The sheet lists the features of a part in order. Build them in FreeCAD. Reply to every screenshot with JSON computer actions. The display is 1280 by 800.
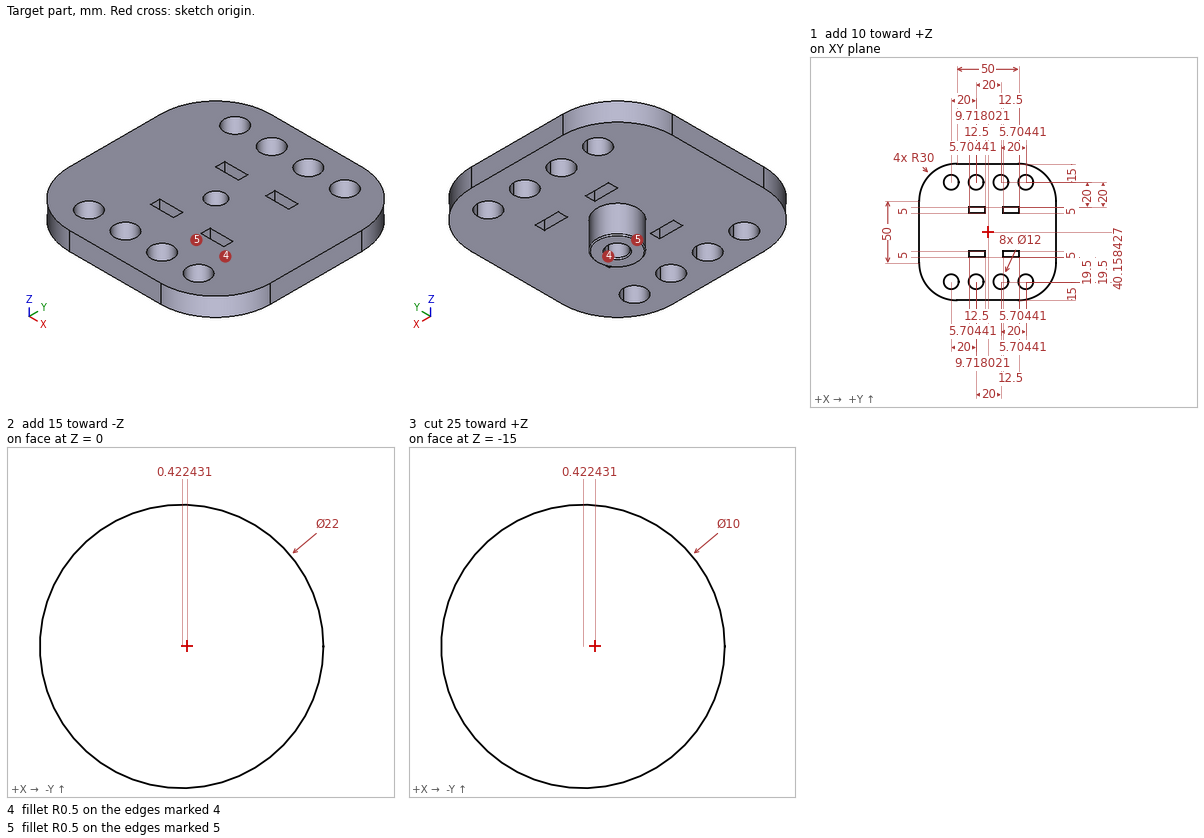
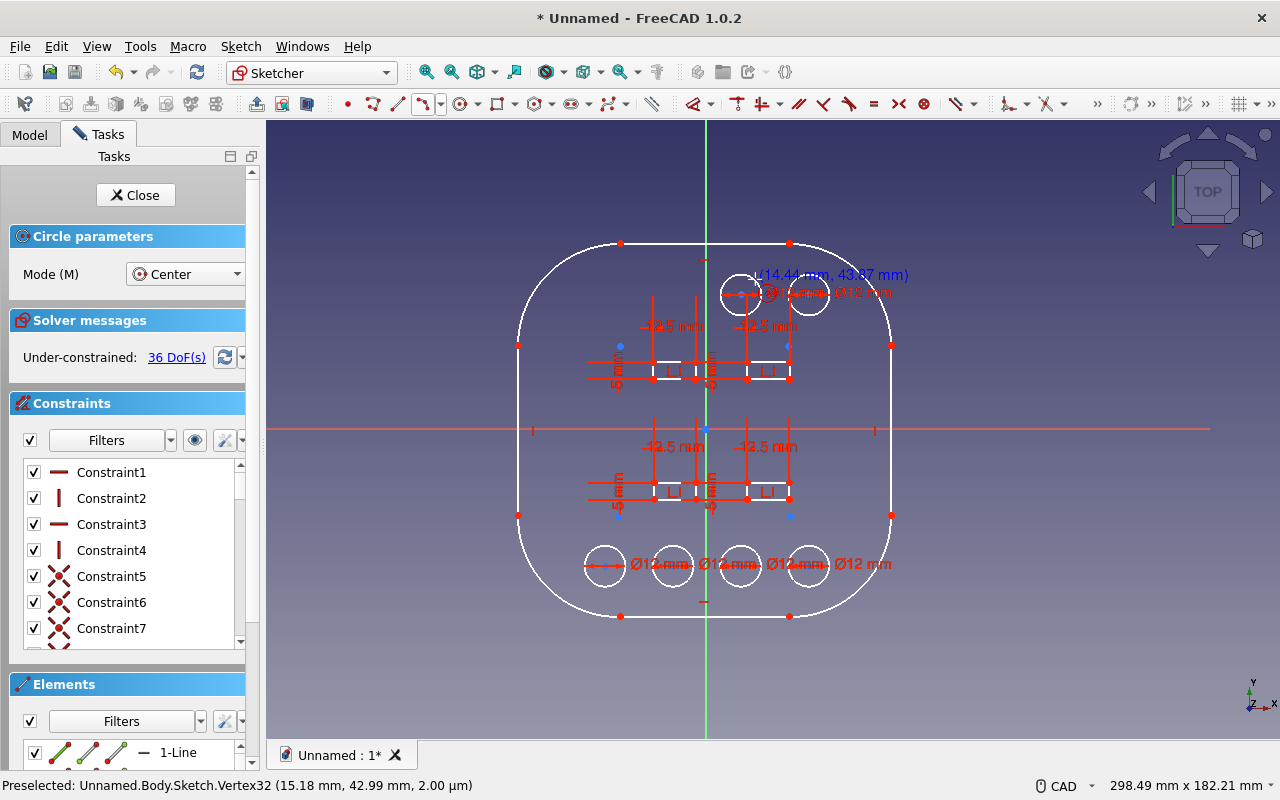
{"action": "left_click", "coordinate": [673, 294]}
{"action": "mouse_move", "coordinate": [687, 279]}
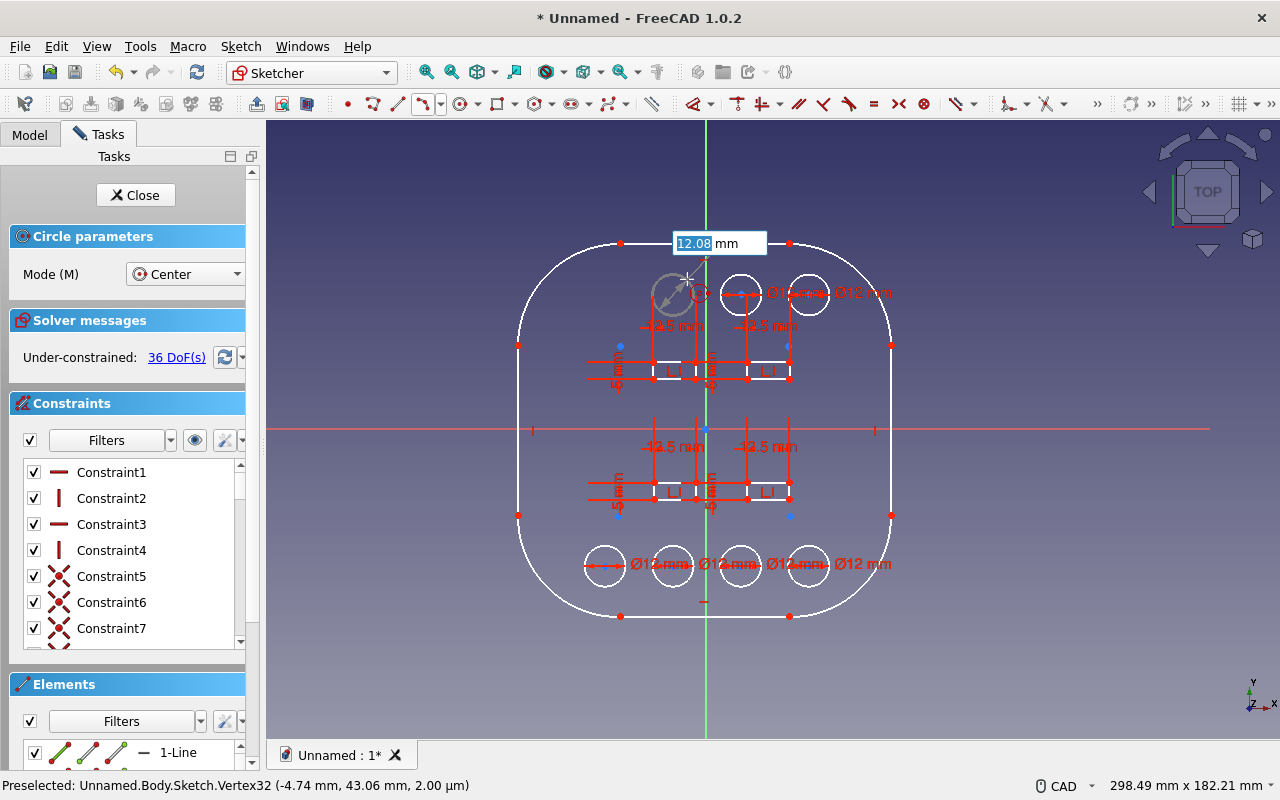
{"action": "type", "text": "12"}
{"action": "key", "text": "Return"}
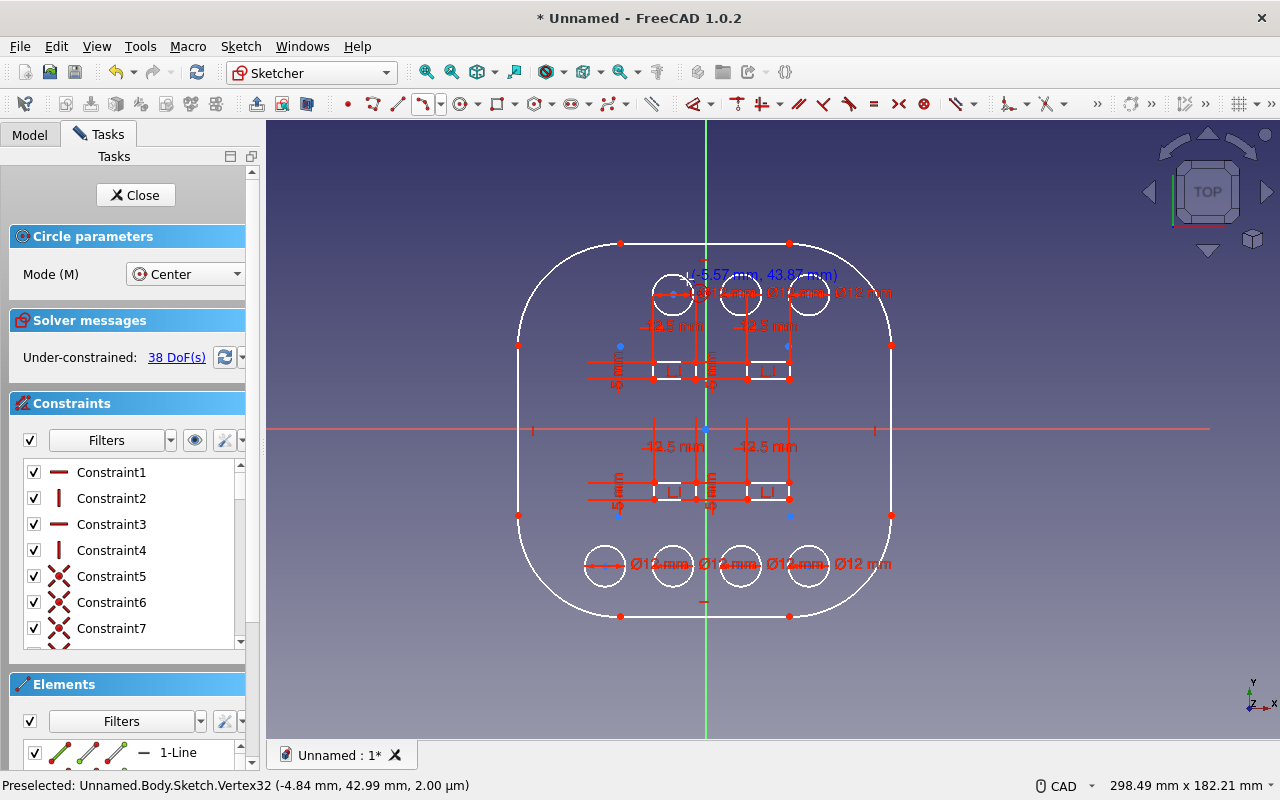
{"action": "left_click", "coordinate": [605, 294]}
{"action": "mouse_move", "coordinate": [619, 279]}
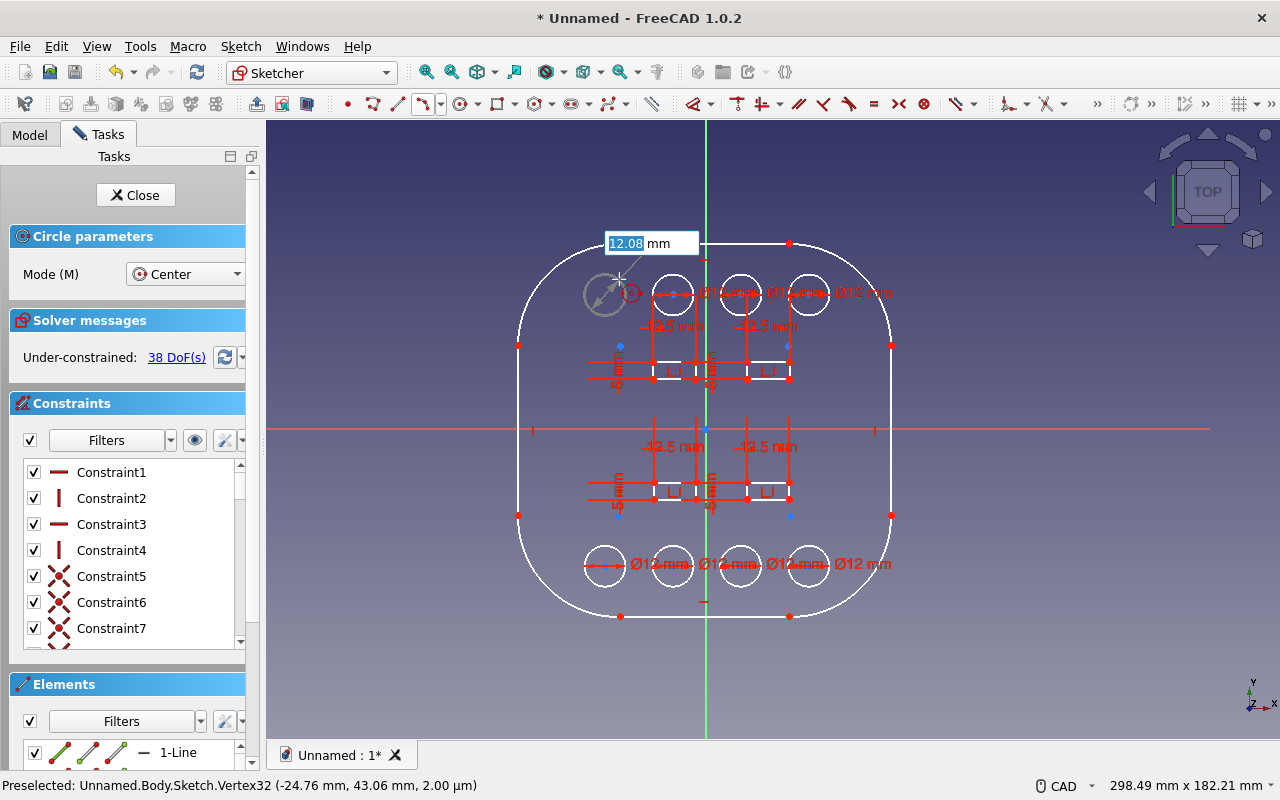
{"action": "type", "text": "12"}
{"action": "key", "text": "Return"}
{"action": "key", "text": "Escape"}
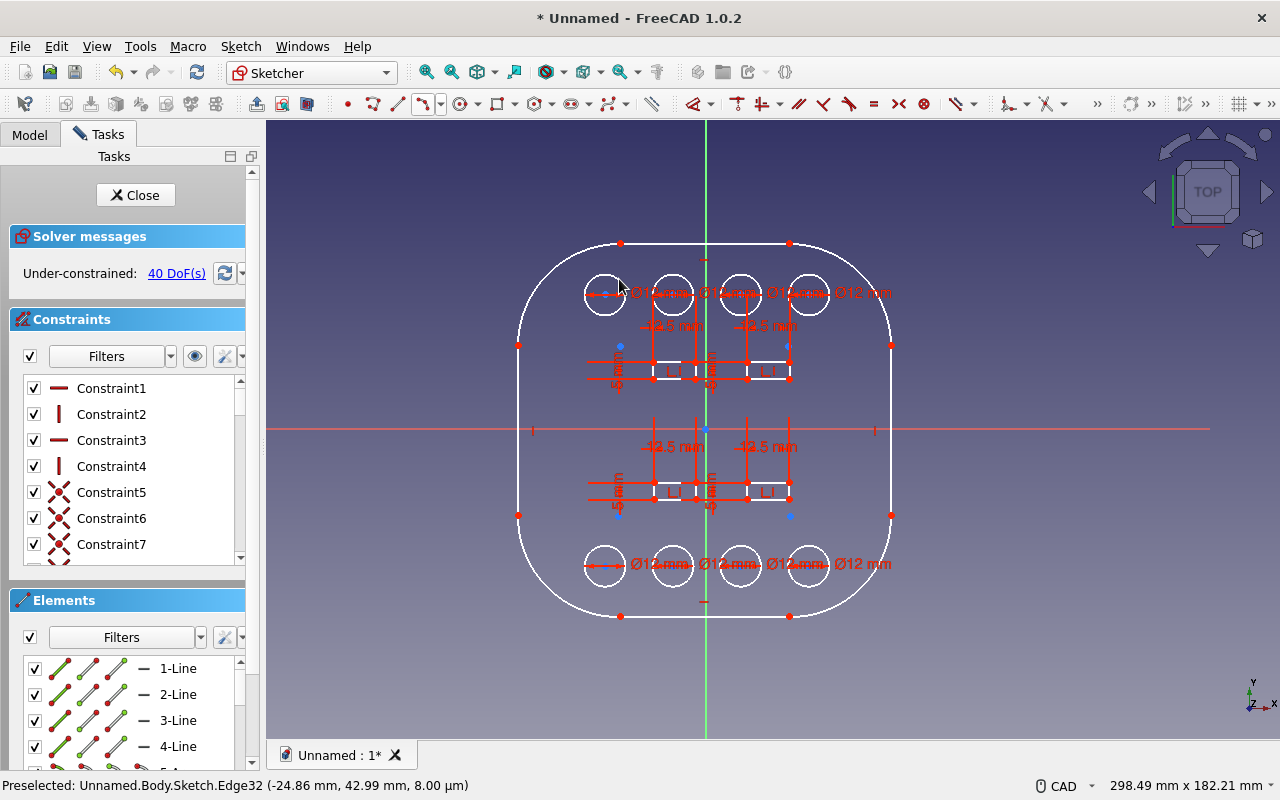
{"action": "left_click", "coordinate": [738, 244]}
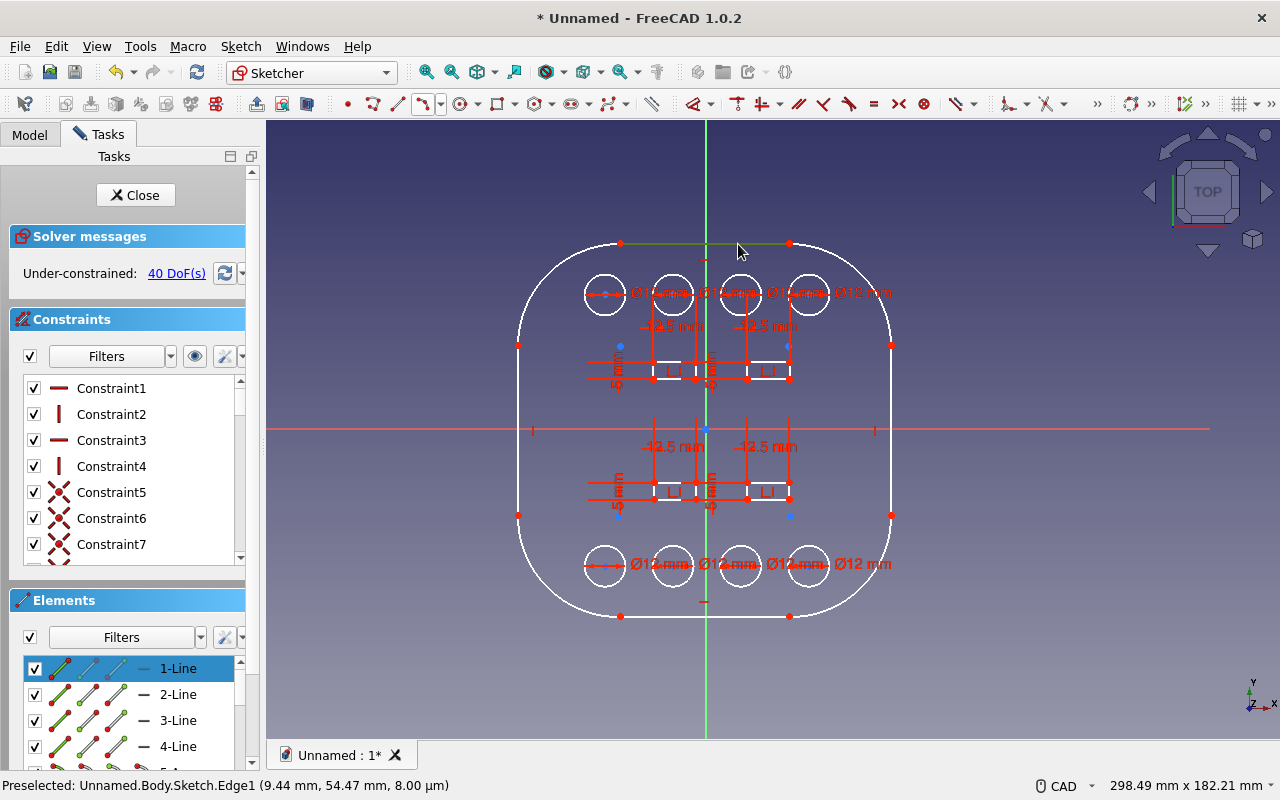
{"action": "left_click", "coordinate": [574, 255]}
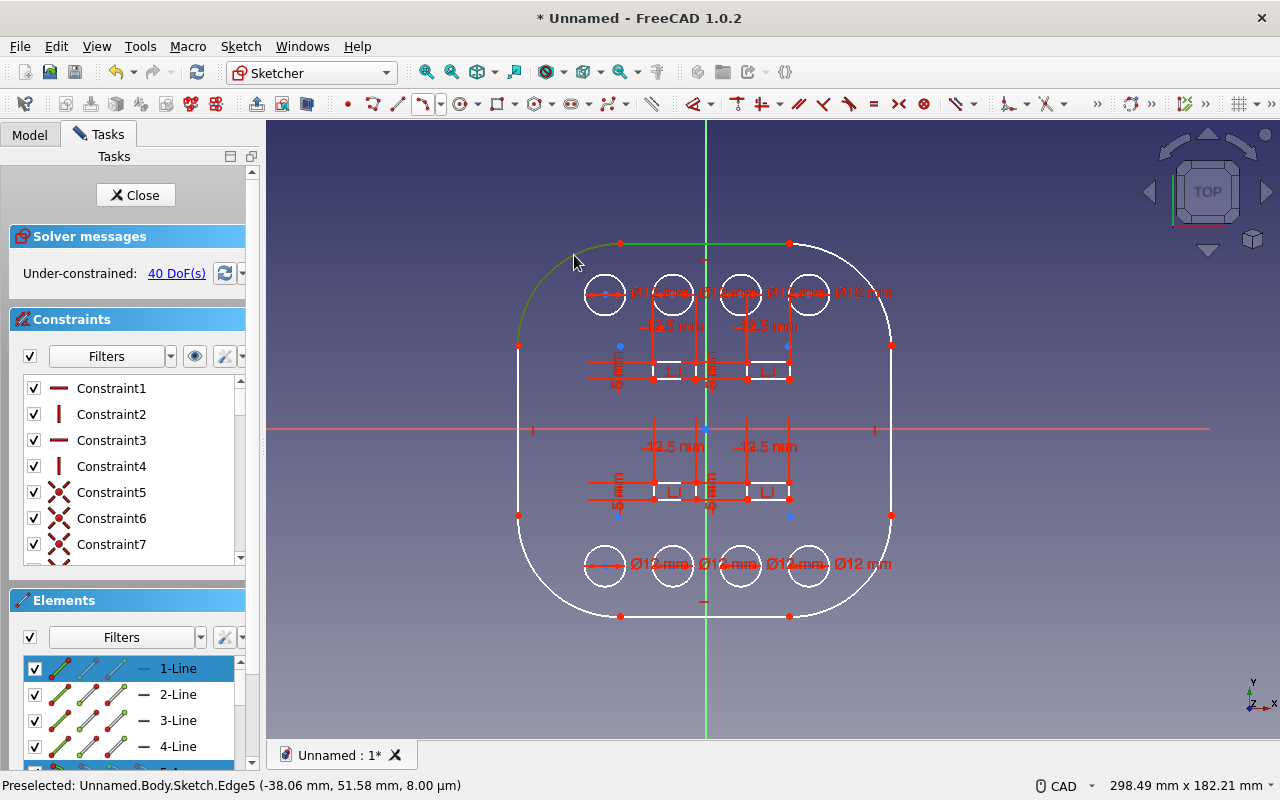
{"action": "left_click", "coordinate": [849, 104]}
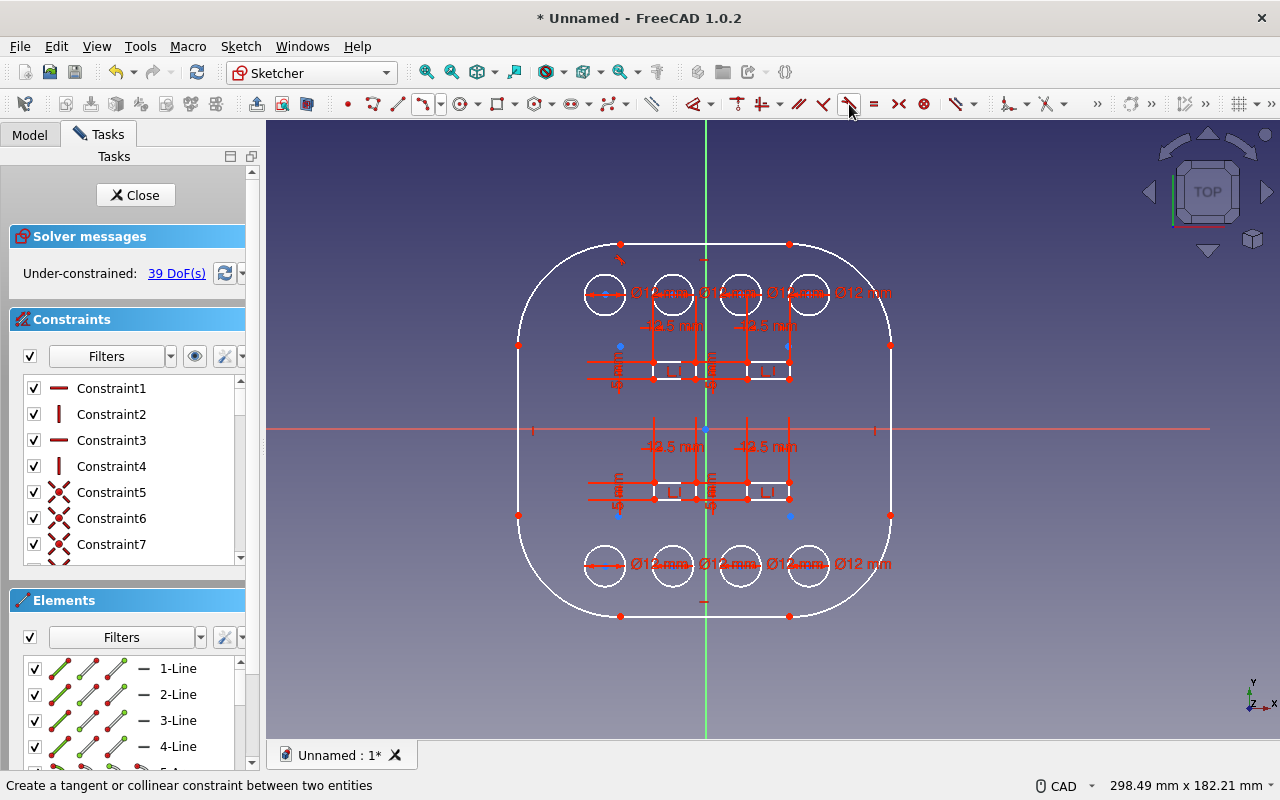
{"action": "left_click", "coordinate": [738, 244]}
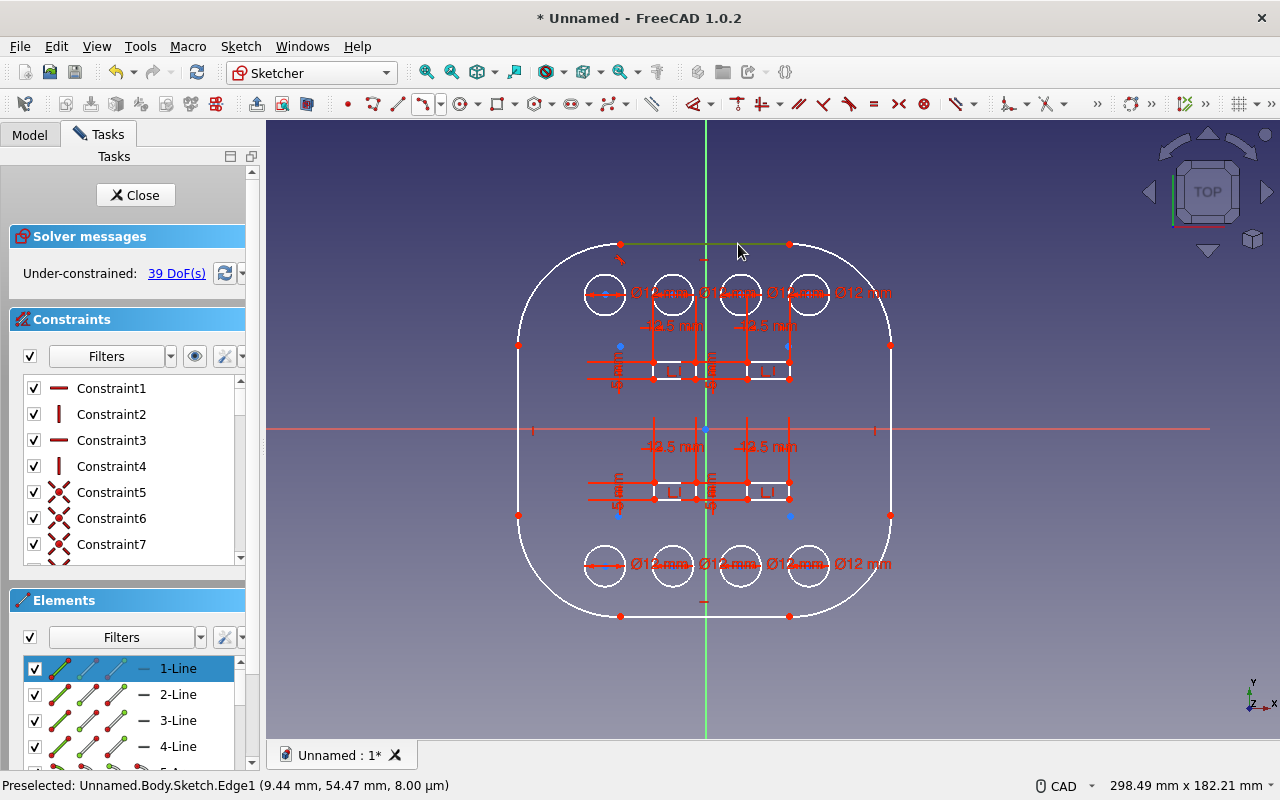
{"action": "left_click", "coordinate": [880, 300]}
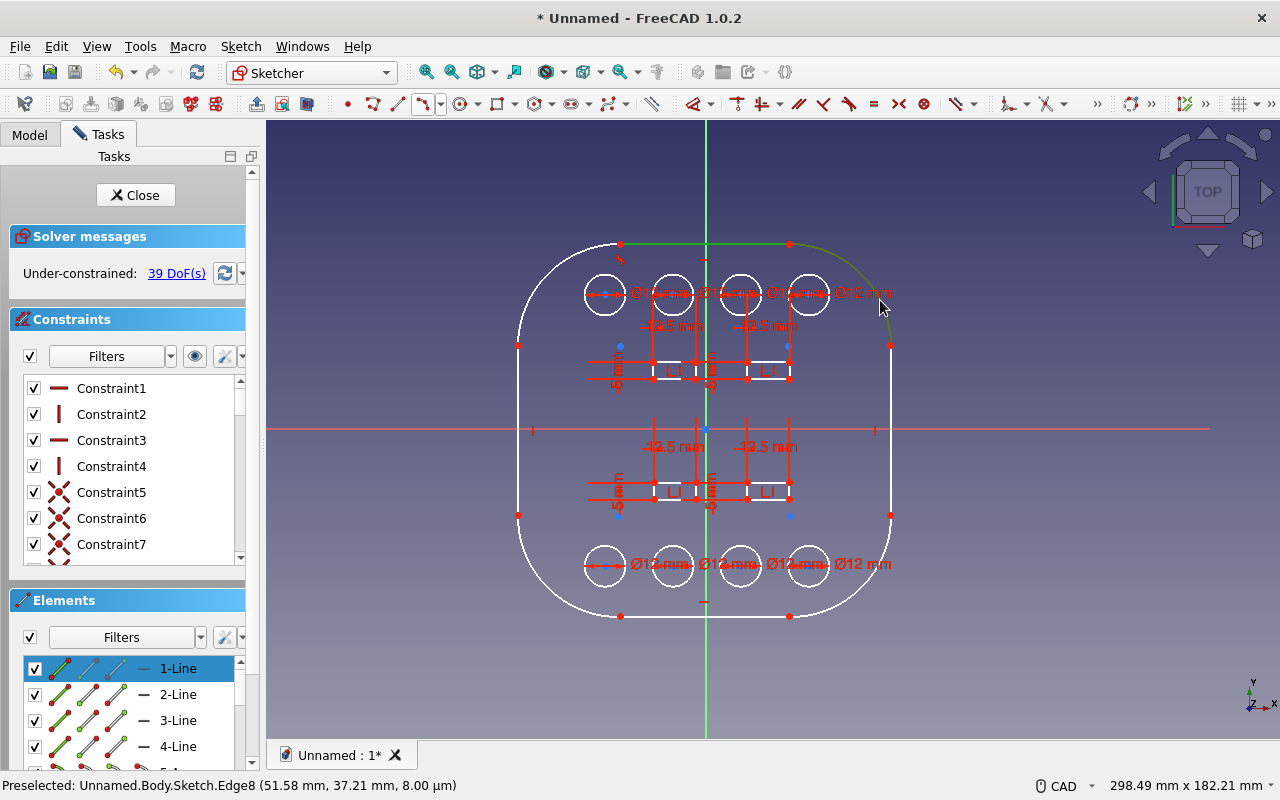
{"action": "key", "text": "t"}